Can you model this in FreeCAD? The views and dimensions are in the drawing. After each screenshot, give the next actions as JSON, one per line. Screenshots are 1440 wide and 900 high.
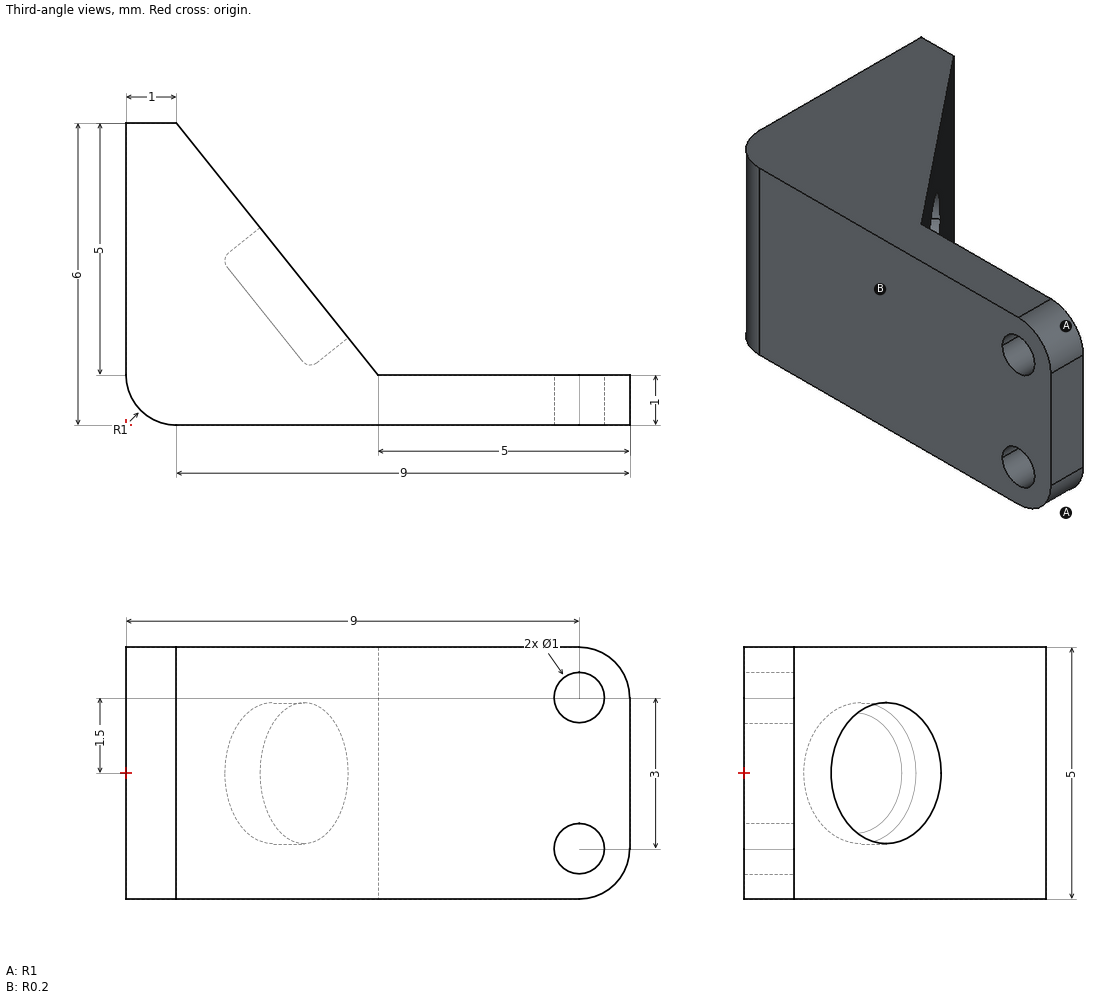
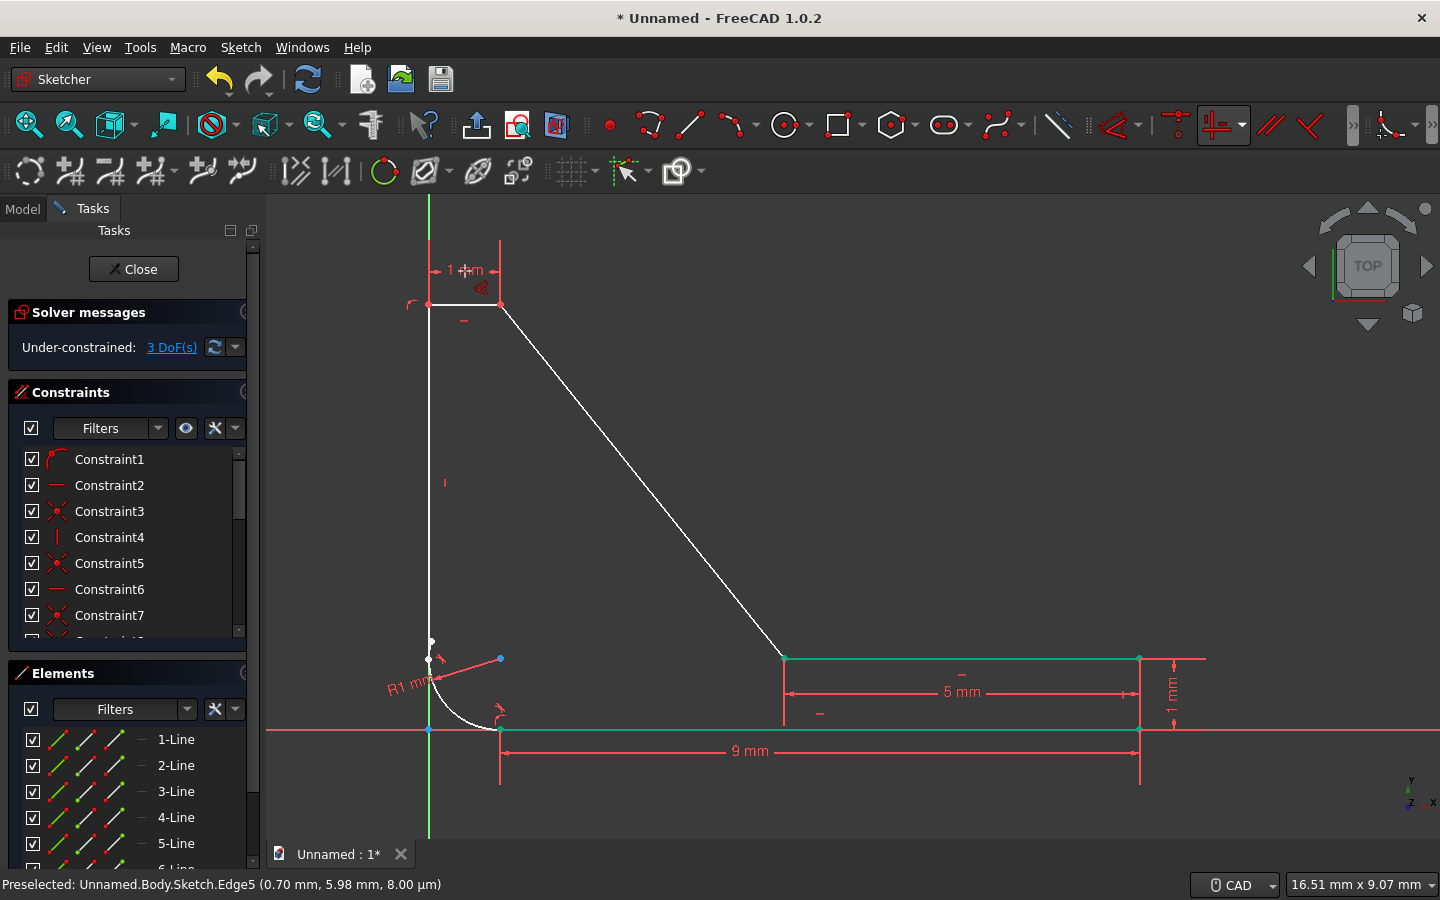
{"action": "left_click", "coordinate": [429, 411]}
{"action": "left_click", "coordinate": [395, 482]}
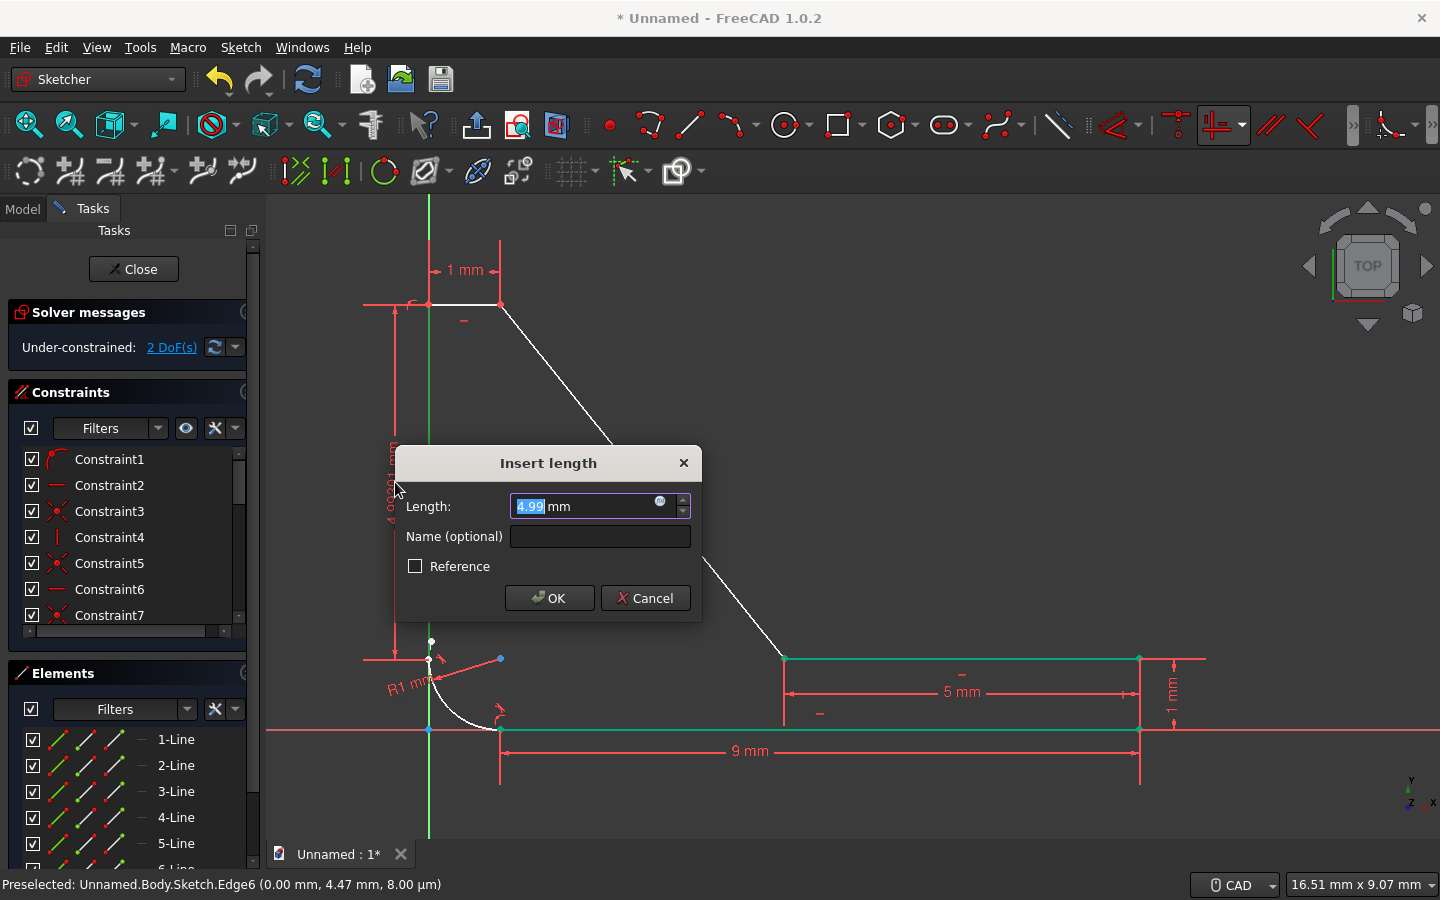
{"action": "type", "text": "5"}
{"action": "key", "text": "Return"}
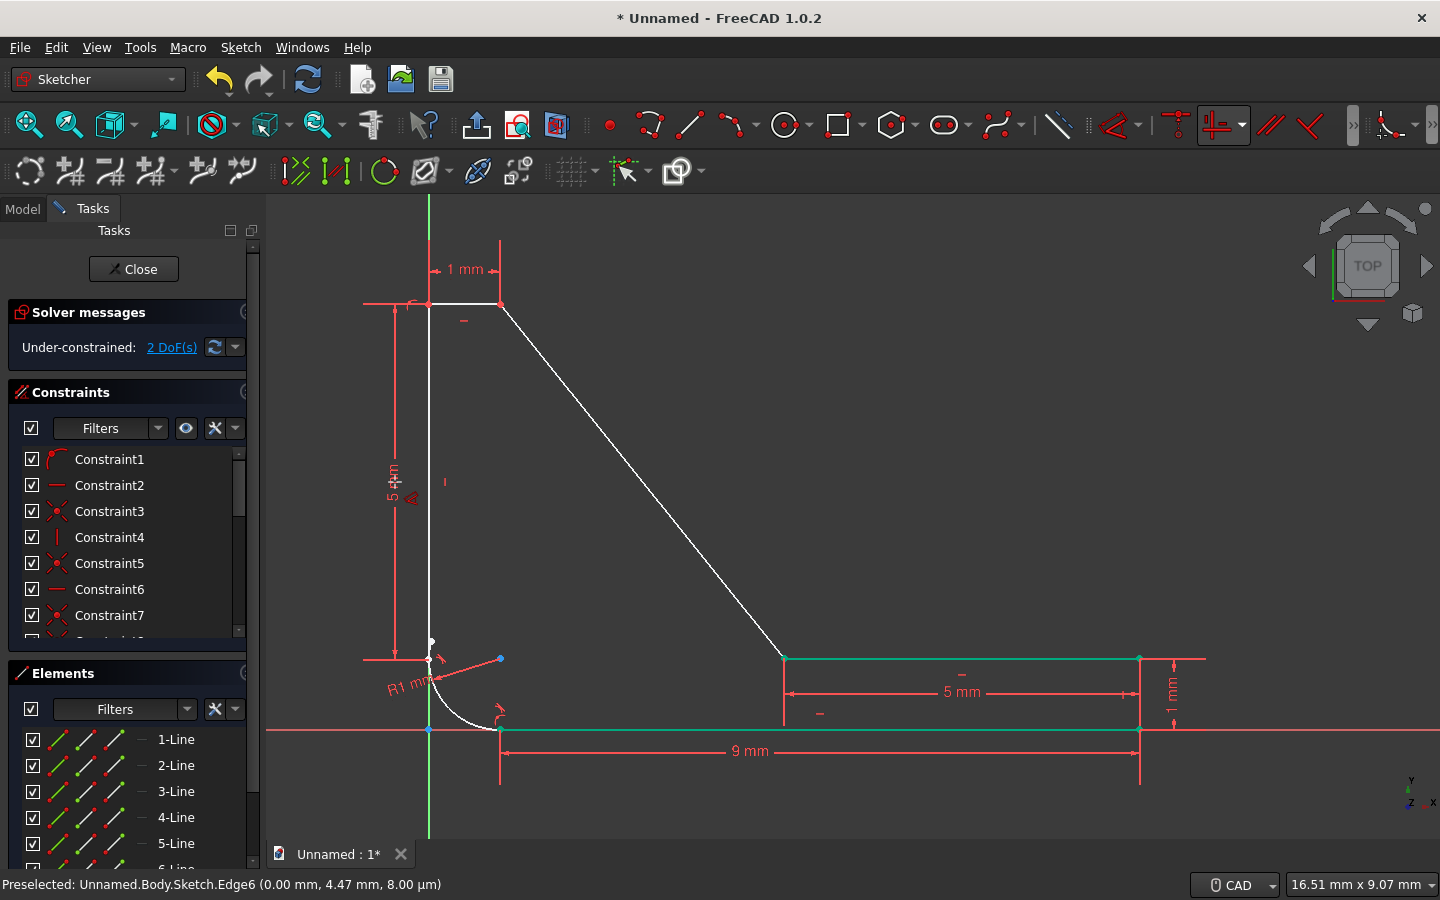
{"action": "left_click", "coordinate": [500, 304]}
{"action": "left_click", "coordinate": [395, 517]}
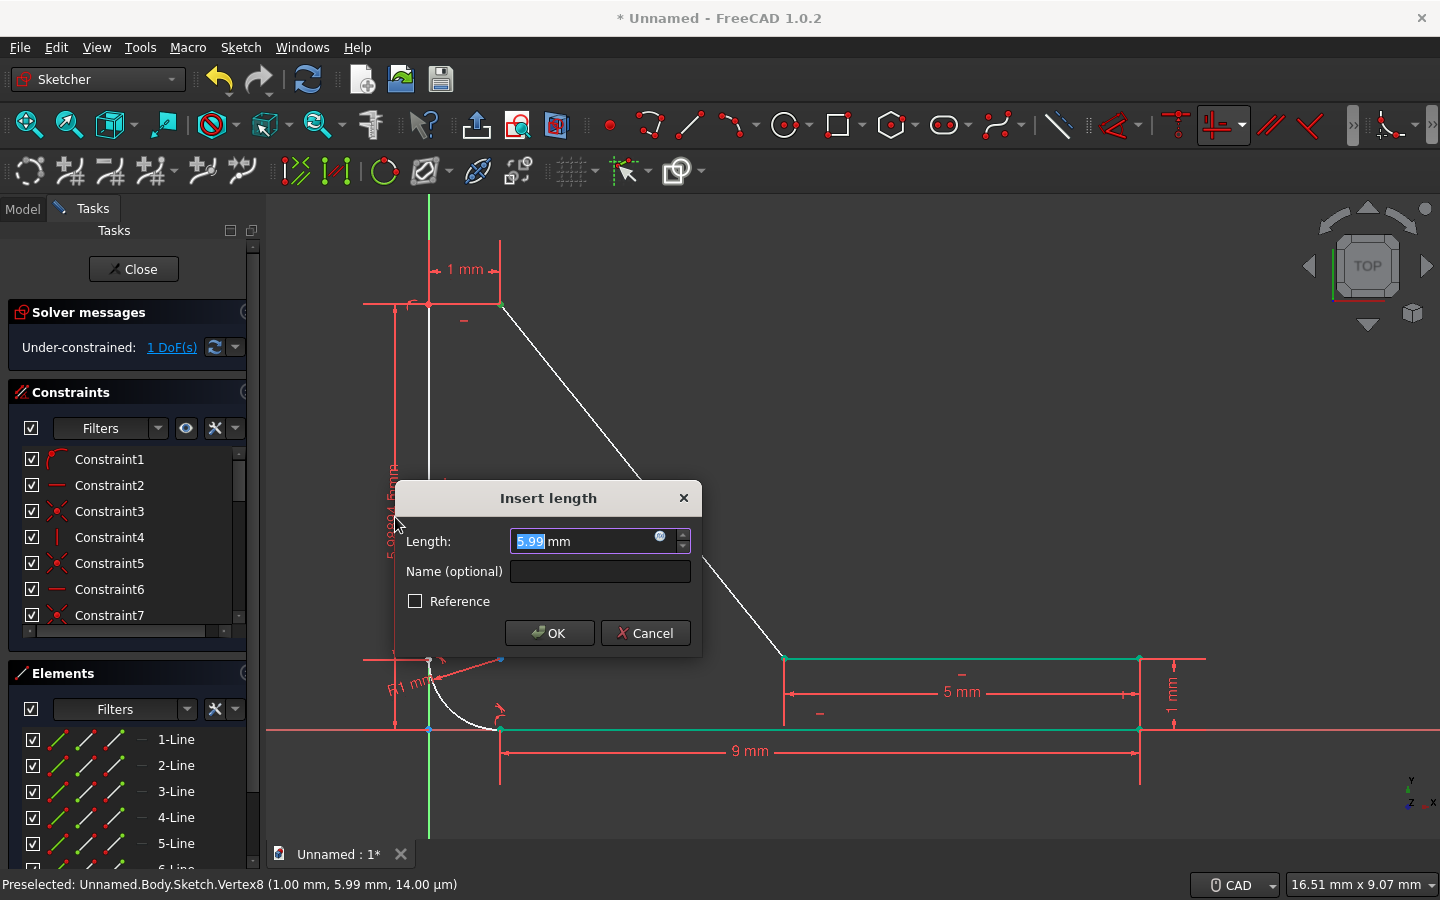
{"action": "type", "text": "6"}
{"action": "key", "text": "Return"}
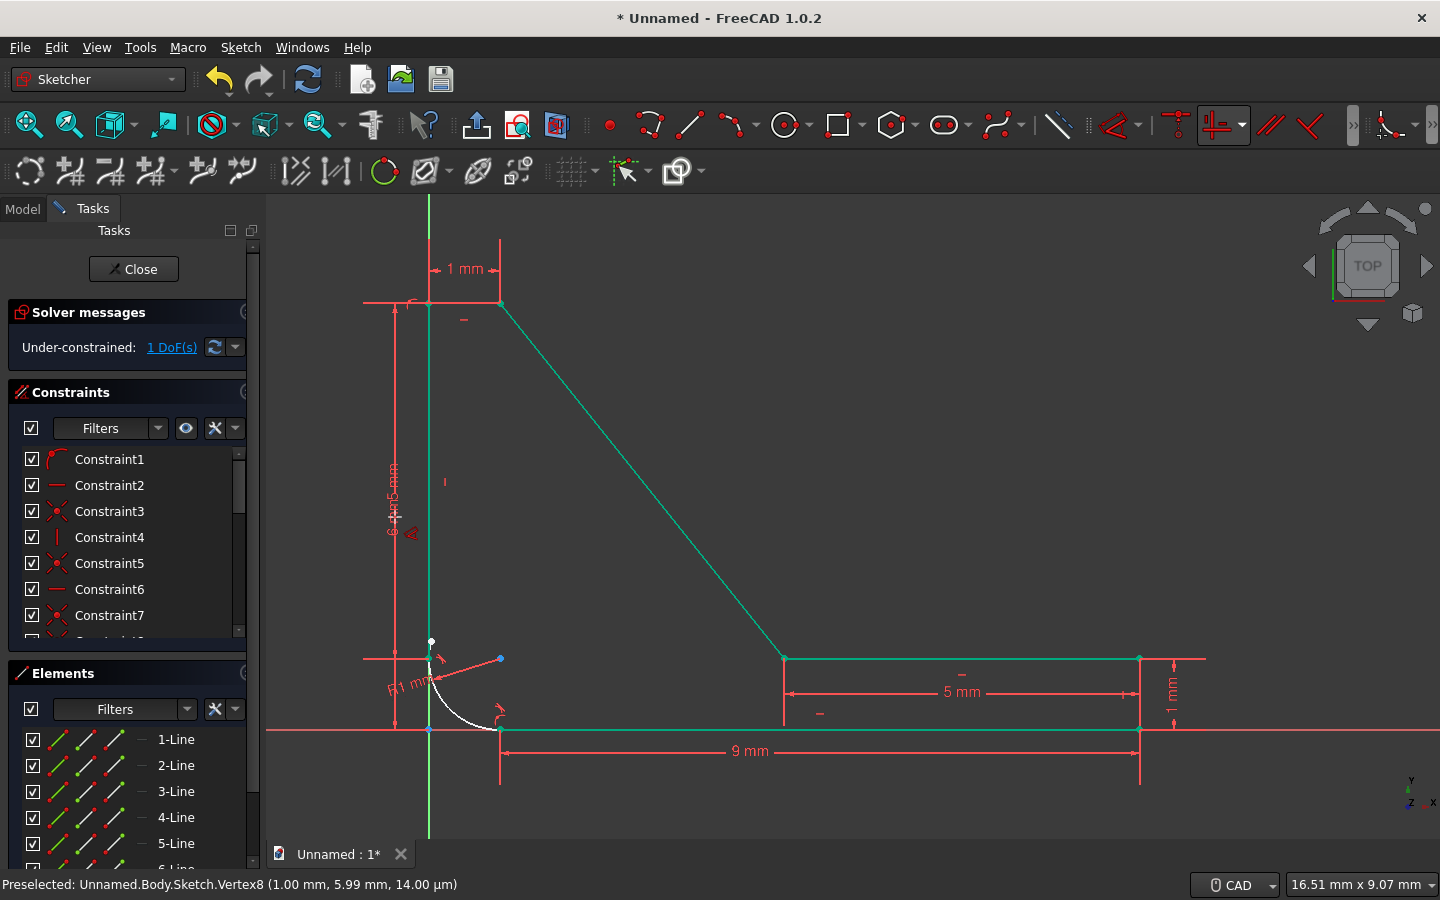
{"action": "left_click", "coordinate": [431, 641]}
{"action": "left_click", "coordinate": [395, 665]}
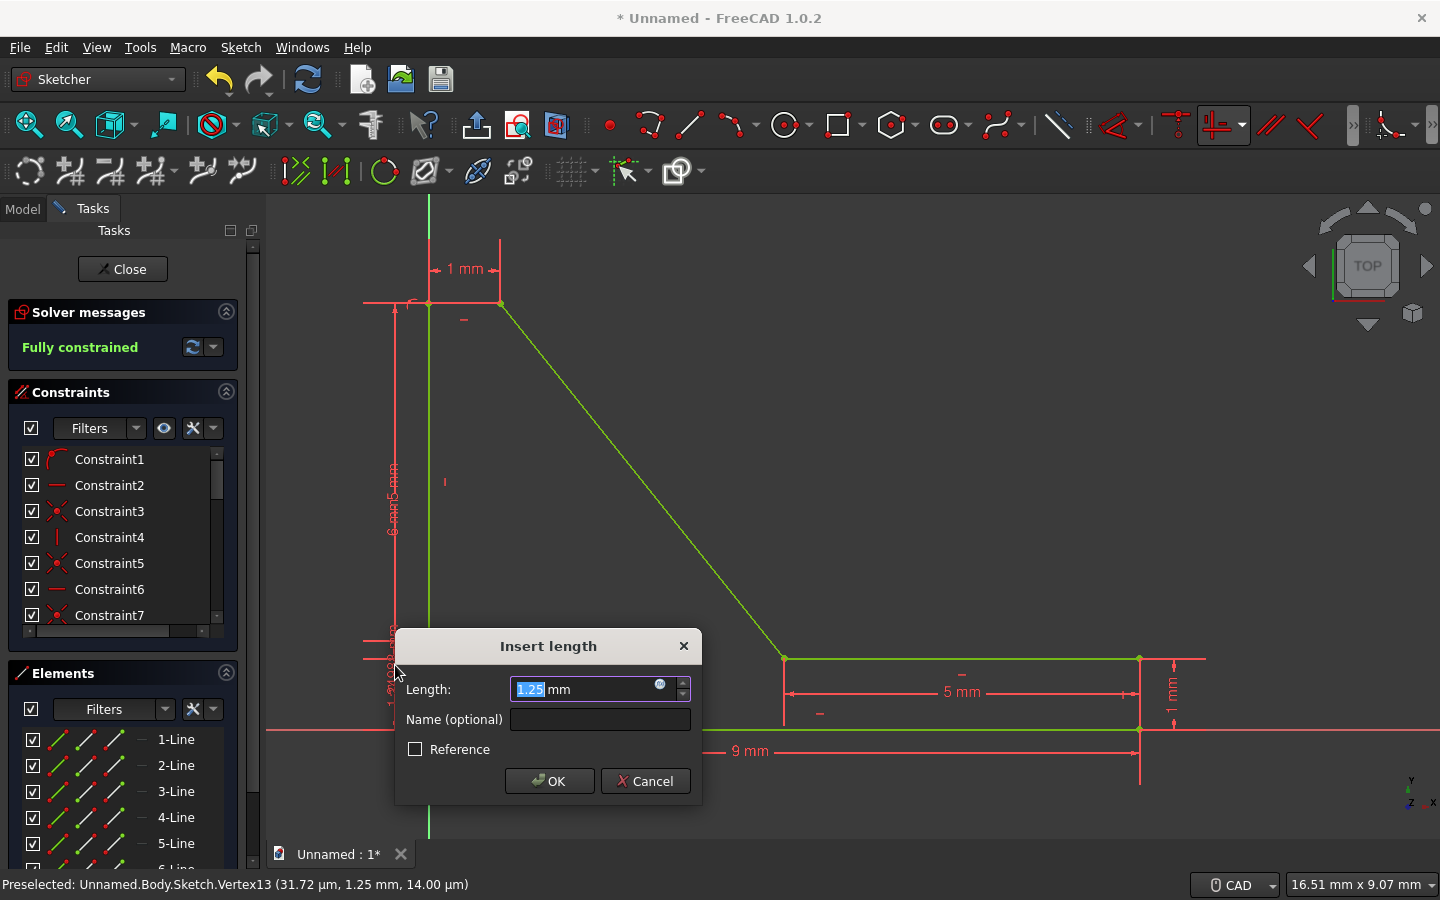
{"action": "type", "text": "1"}
{"action": "key", "text": "Return"}
{"action": "key", "text": "Escape"}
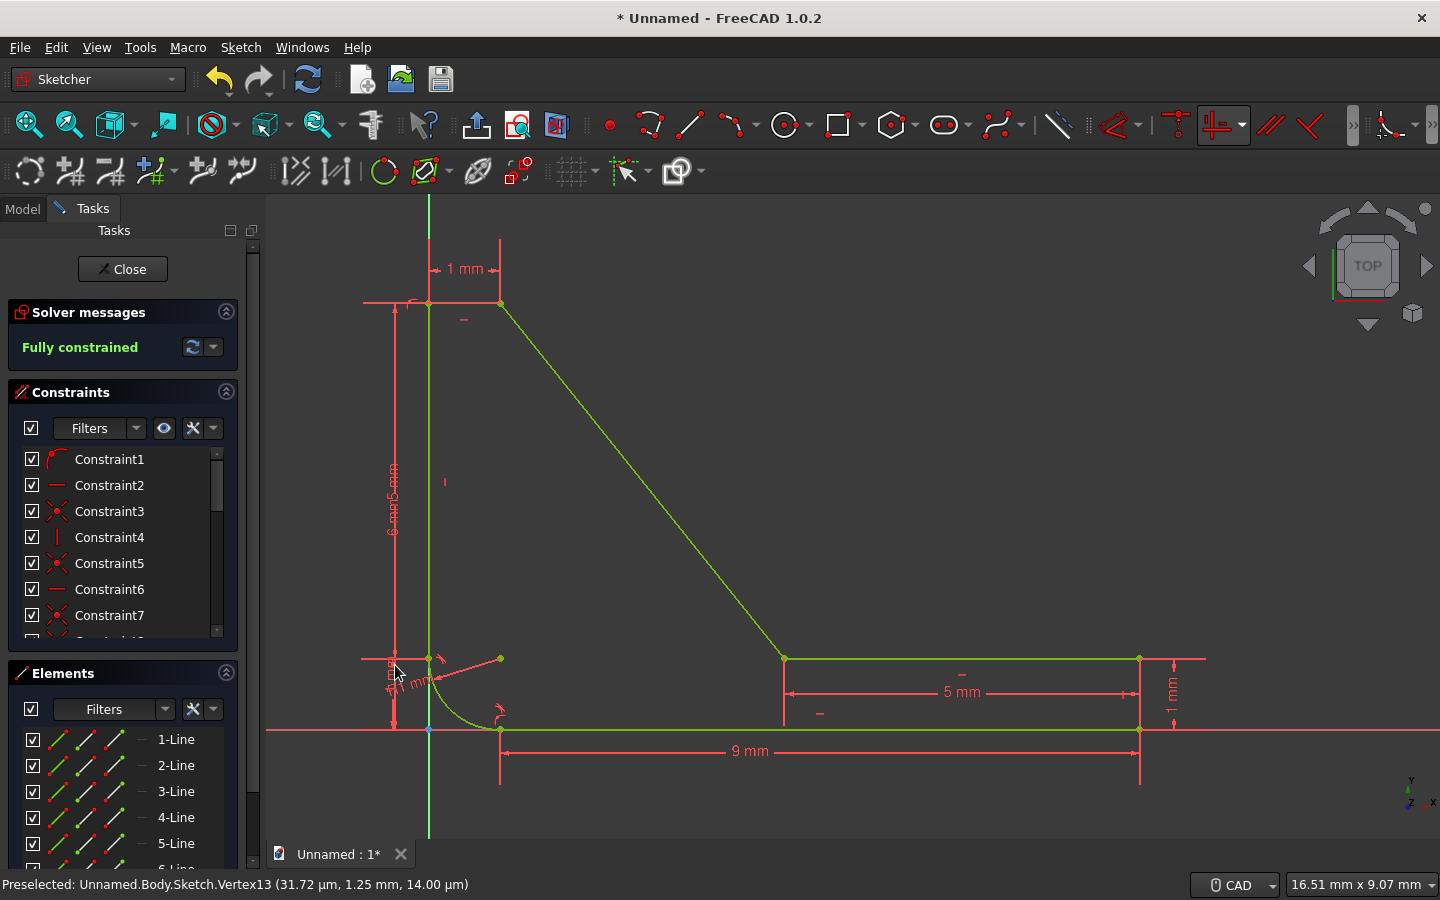
{"action": "left_click", "coordinate": [123, 269]}